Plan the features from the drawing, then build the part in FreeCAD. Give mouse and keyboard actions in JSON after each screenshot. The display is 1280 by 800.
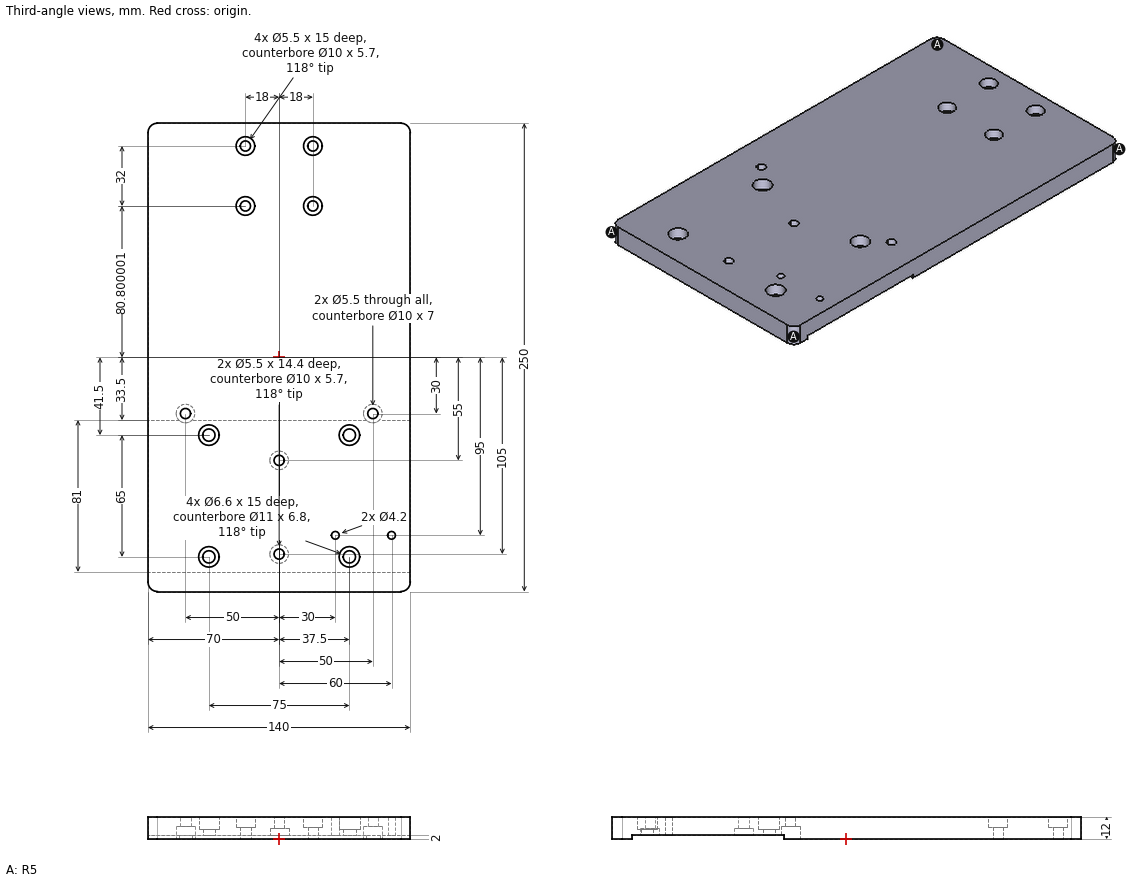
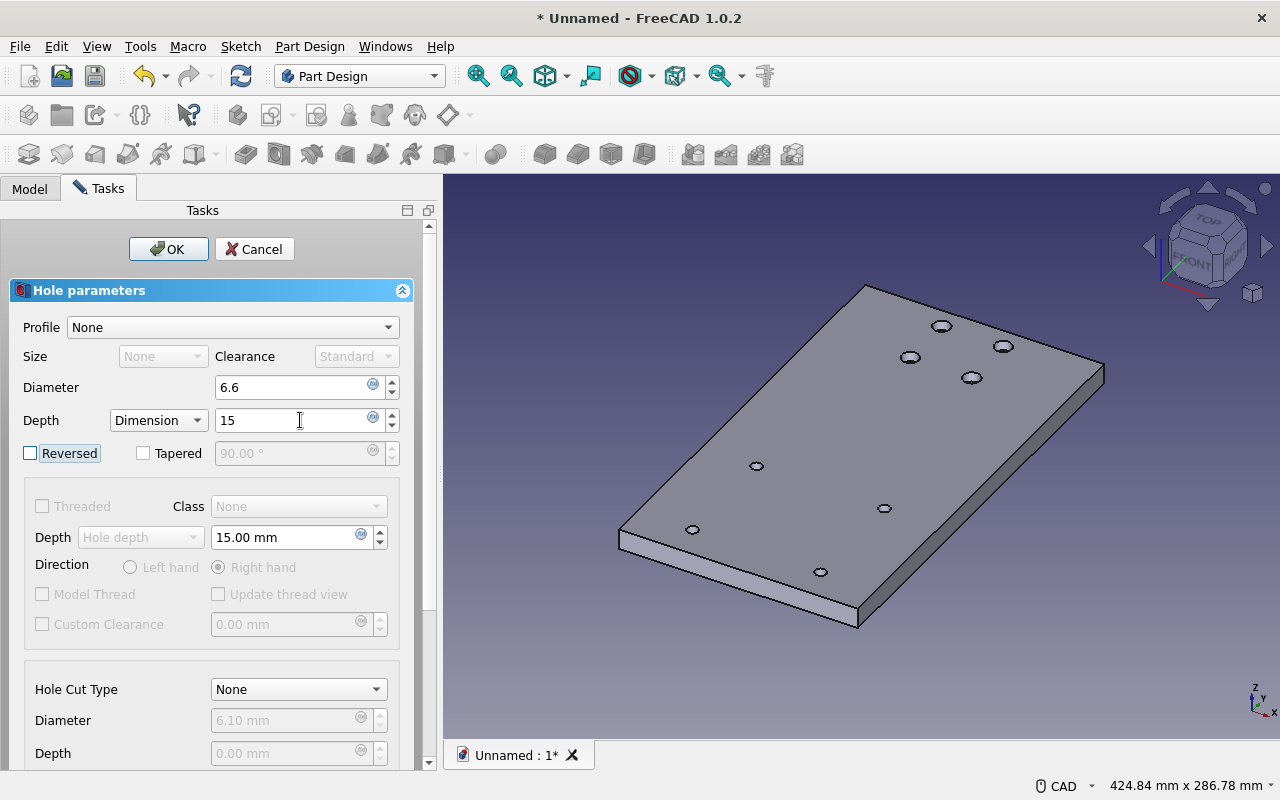
{"action": "left_click", "coordinate": [300, 690]}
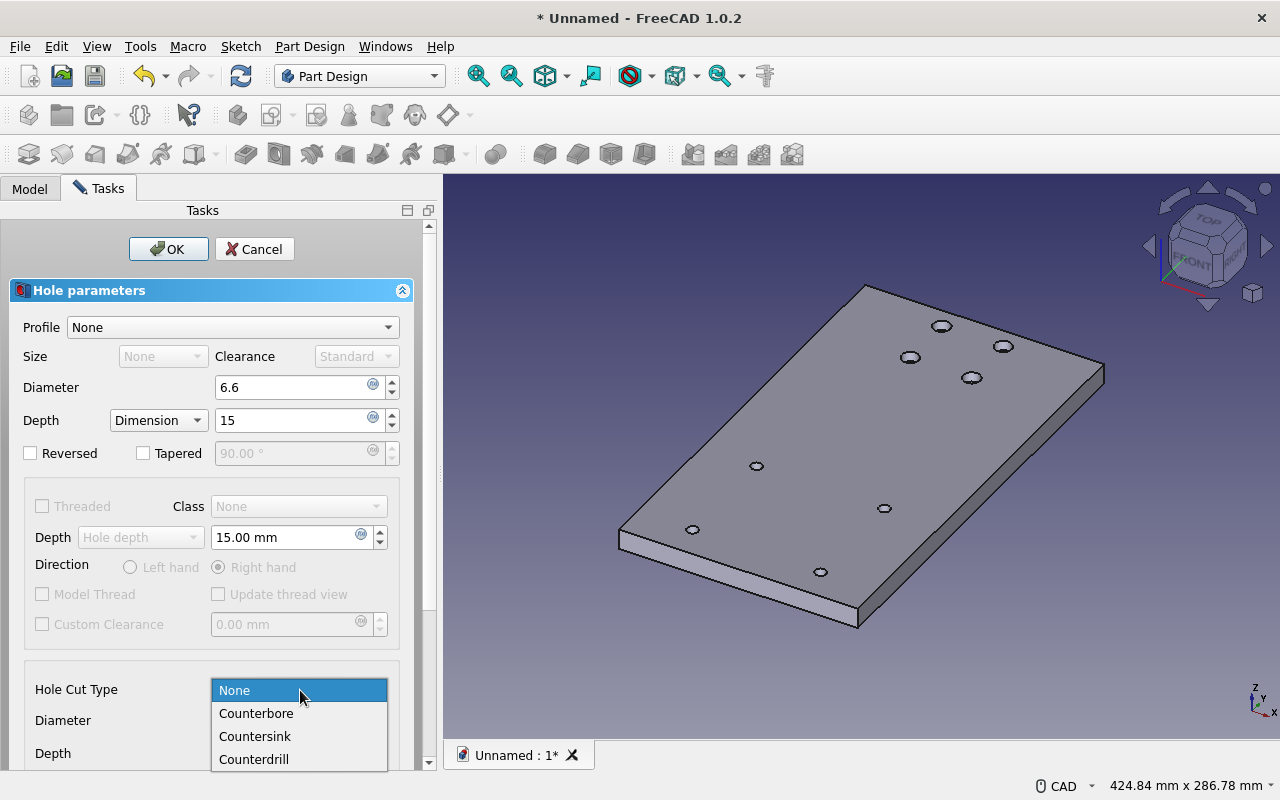
{"action": "left_click", "coordinate": [298, 714]}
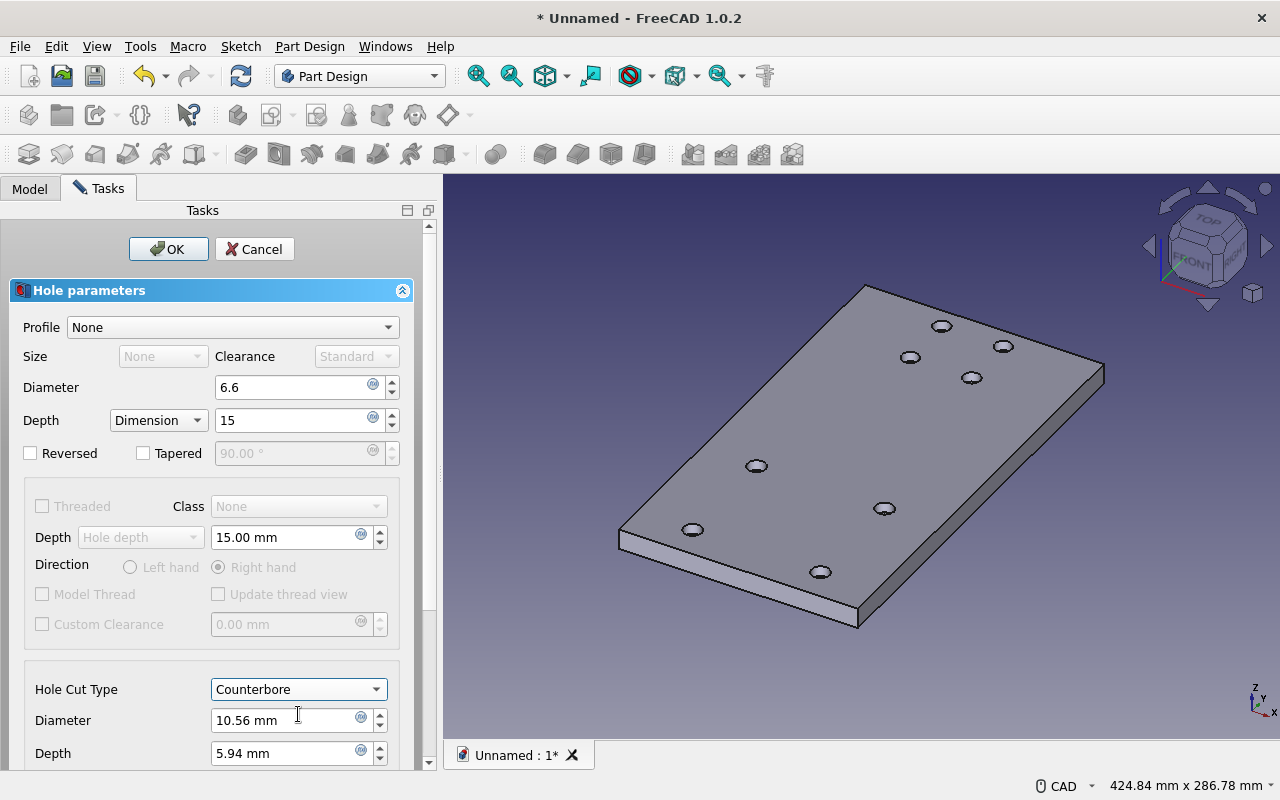
{"action": "triple_click", "coordinate": [292, 720]}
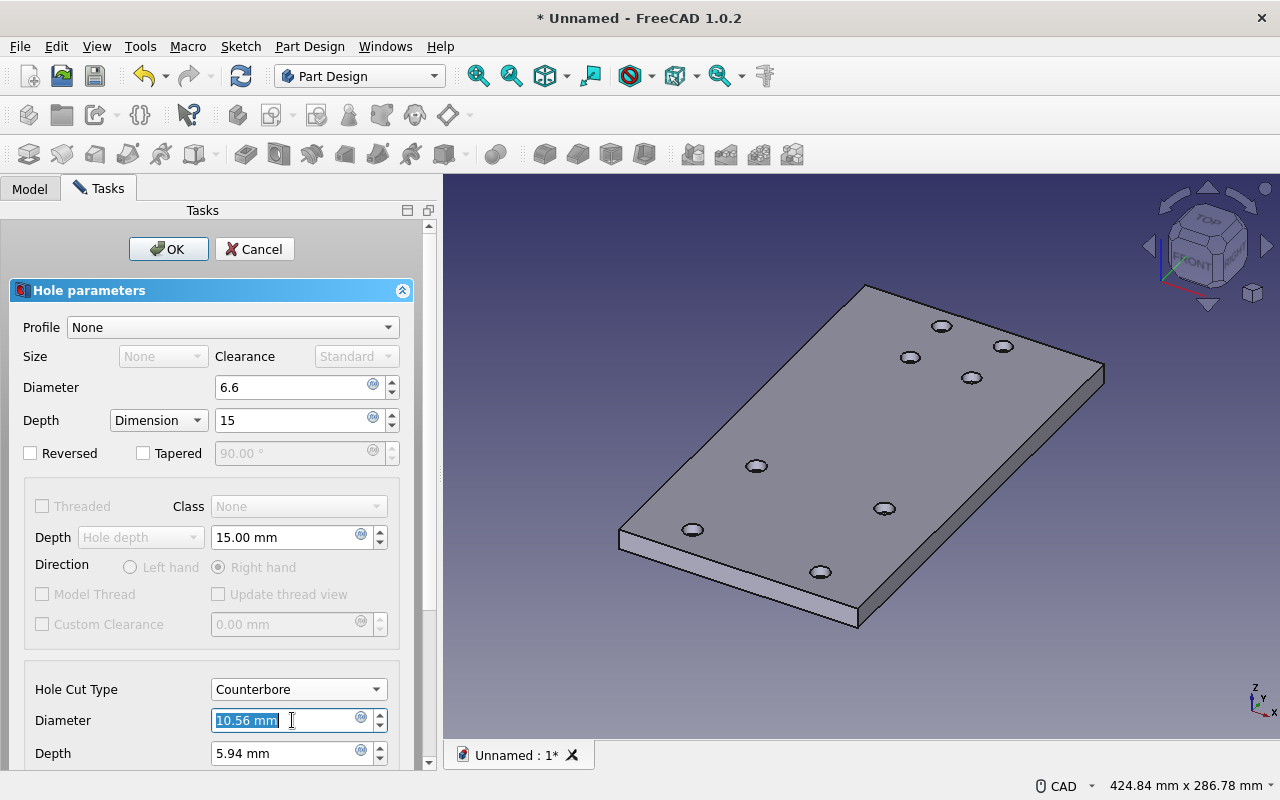
{"action": "type", "text": "11"}
{"action": "key", "text": "Tab"}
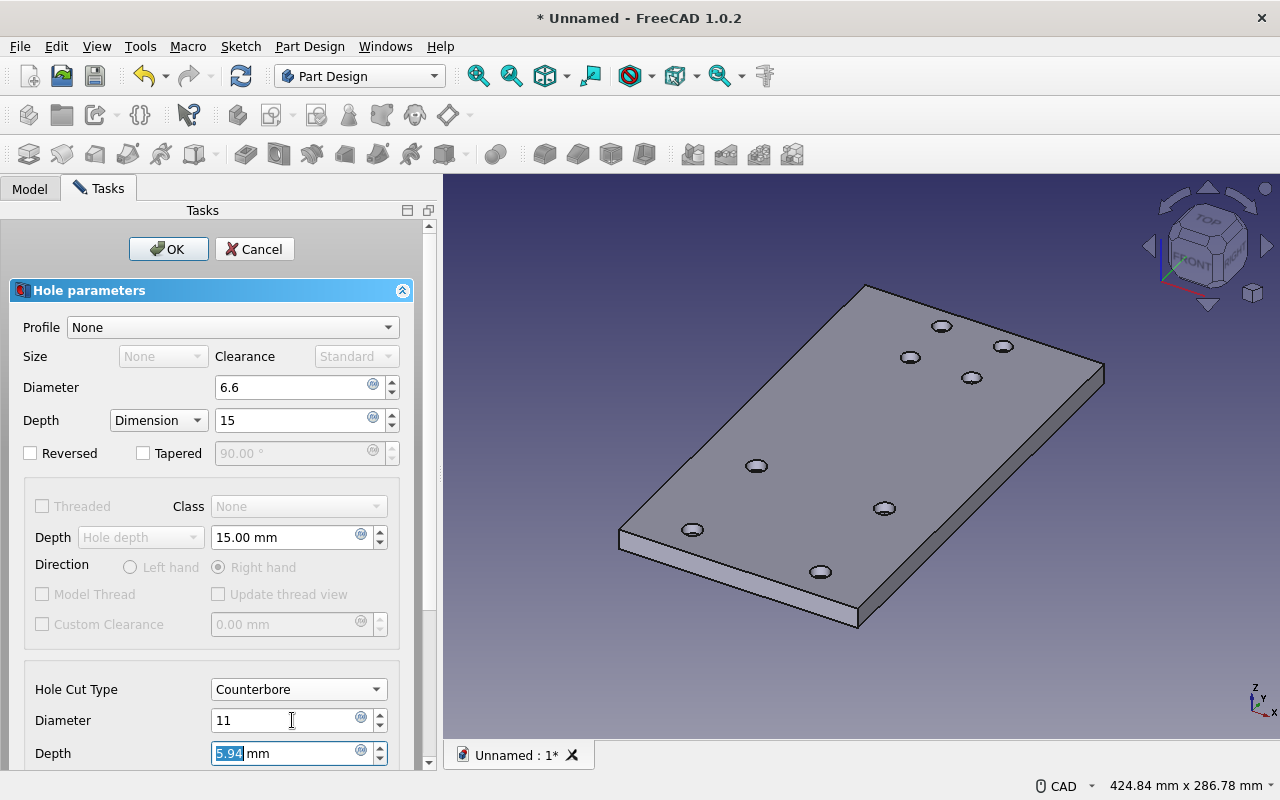
{"action": "type", "text": "6.8"}
{"action": "key", "text": "Tab"}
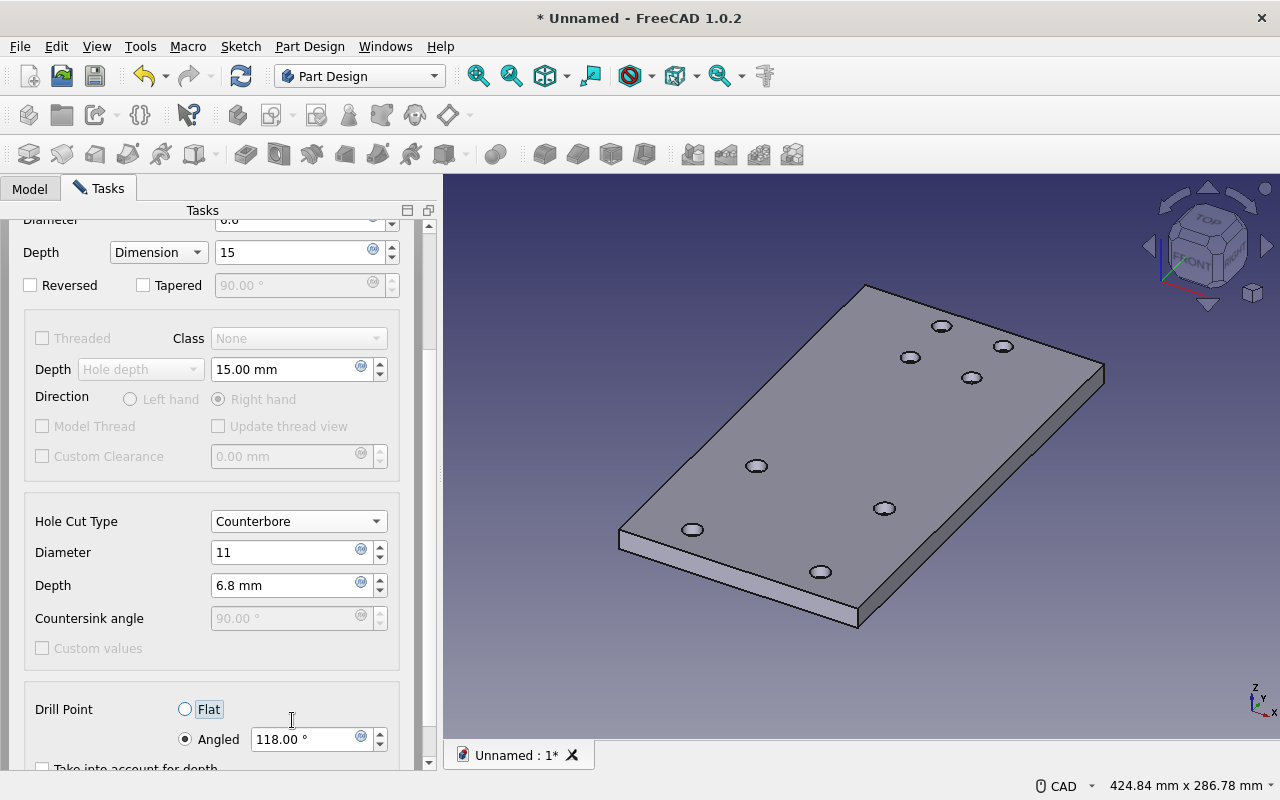
{"action": "scroll", "coordinate": [429, 495], "scroll_direction": "up", "scroll_amount": 4}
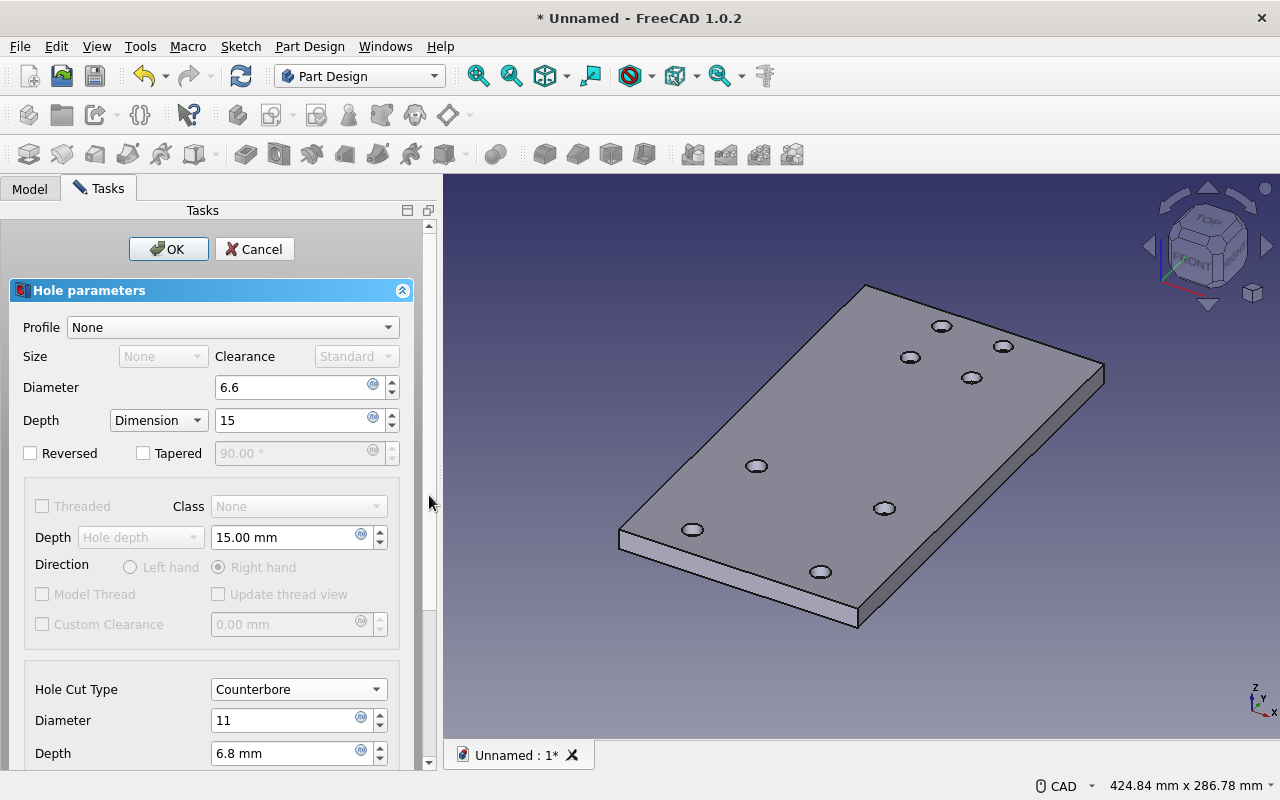
{"action": "left_click", "coordinate": [169, 249]}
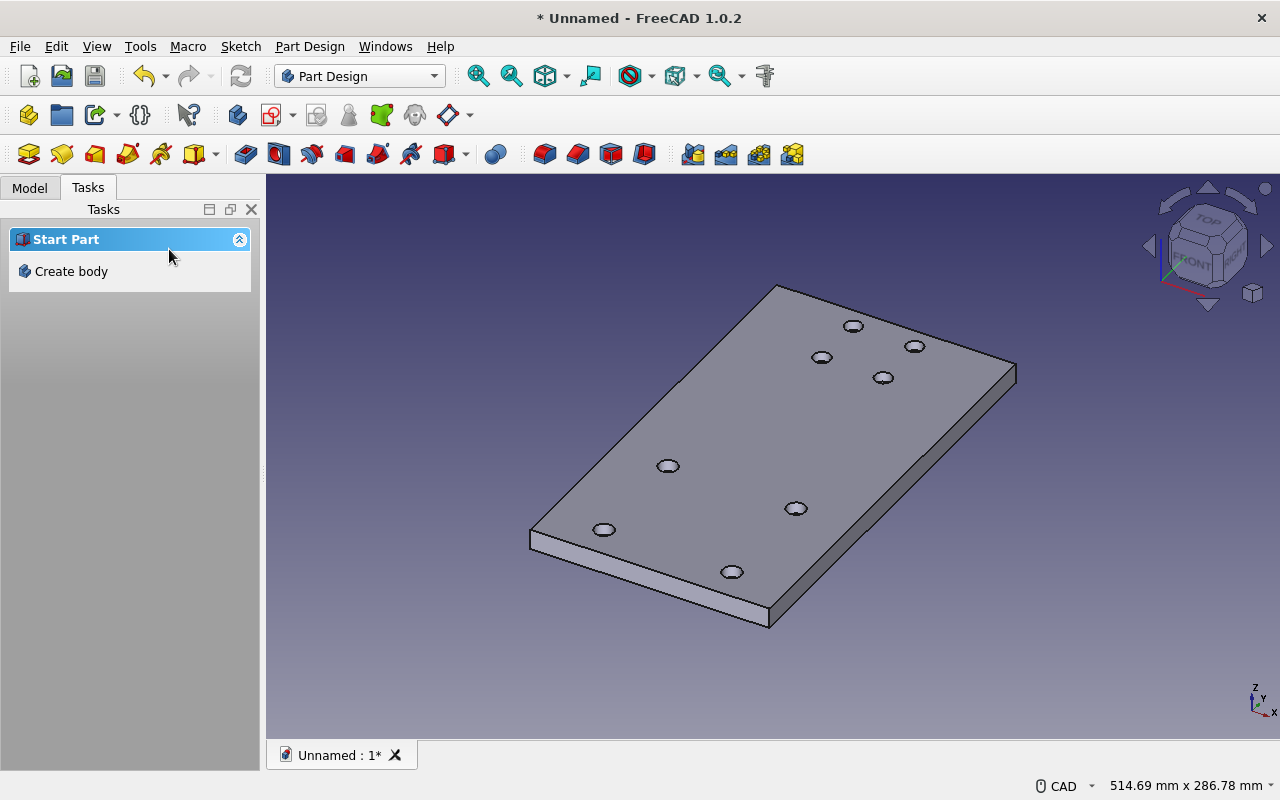
{"action": "left_click", "coordinate": [270, 116]}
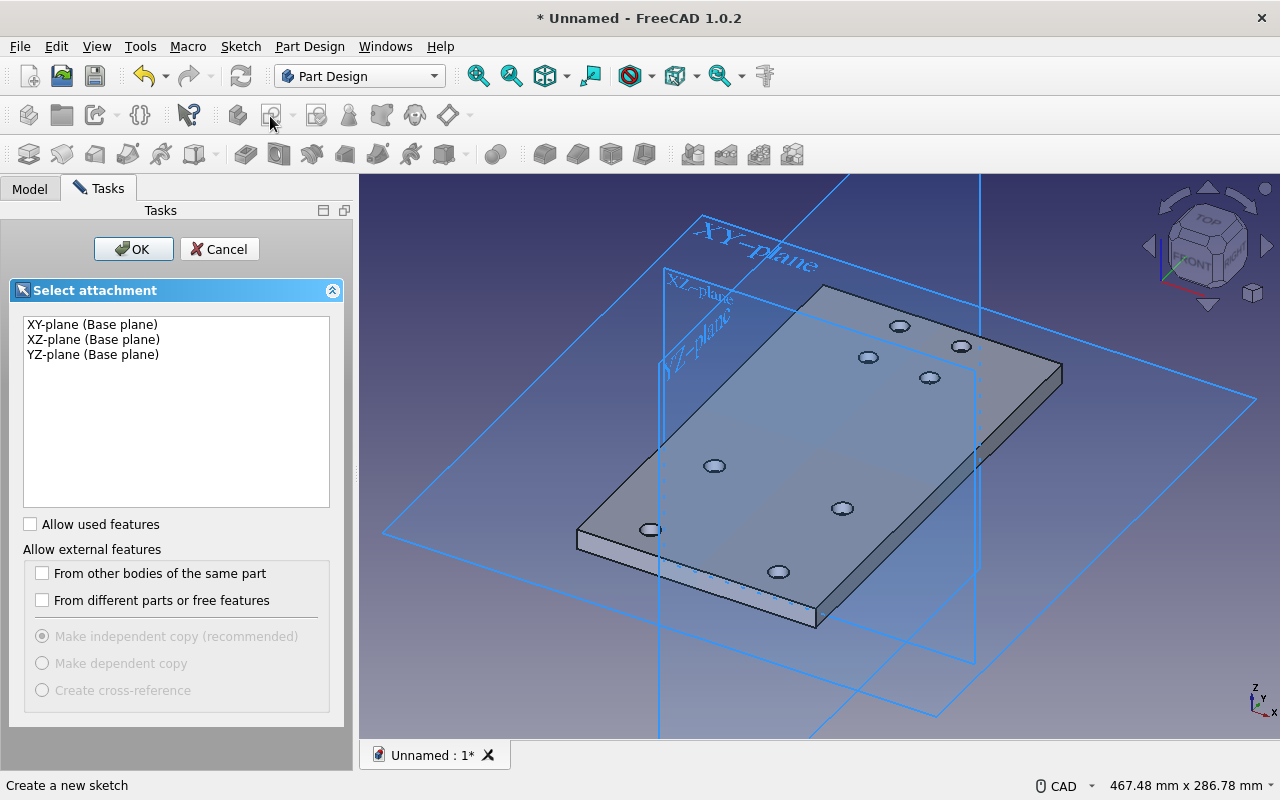
{"action": "left_click", "coordinate": [84, 324]}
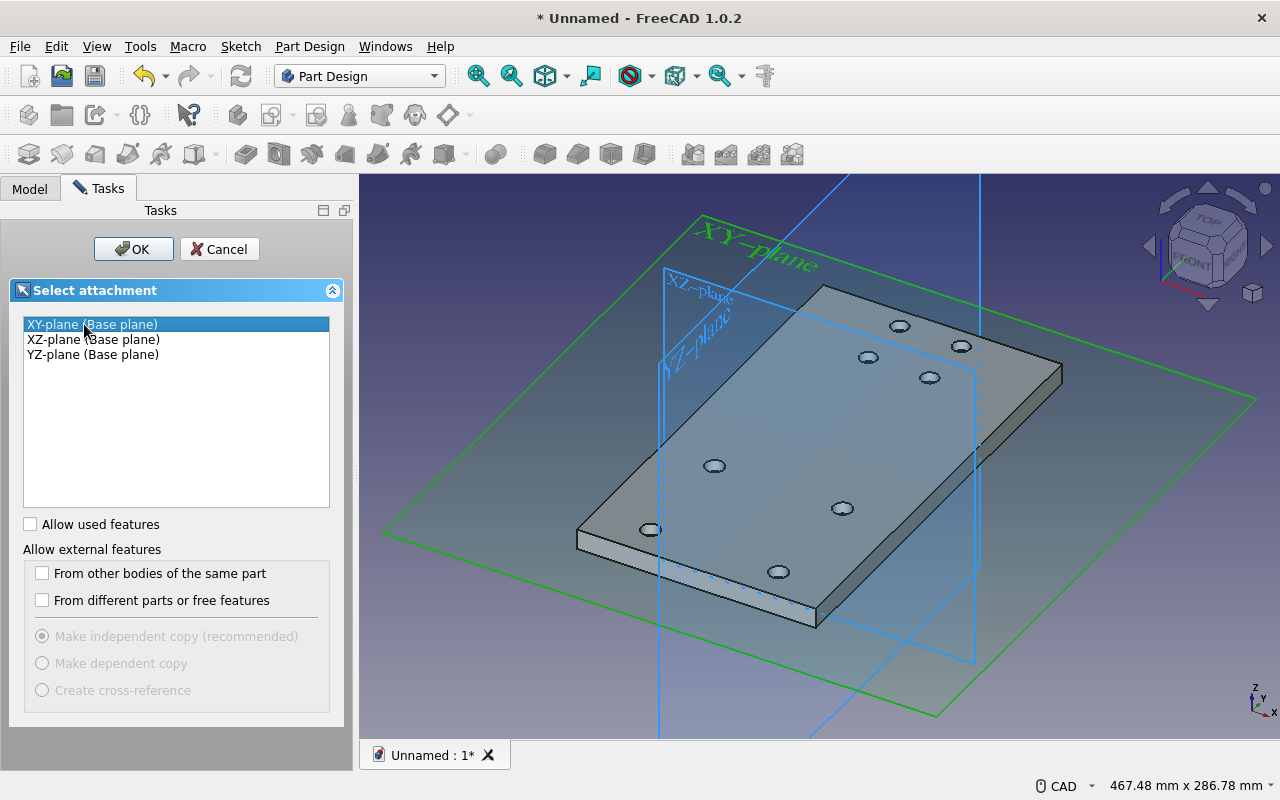
{"action": "left_click", "coordinate": [134, 249]}